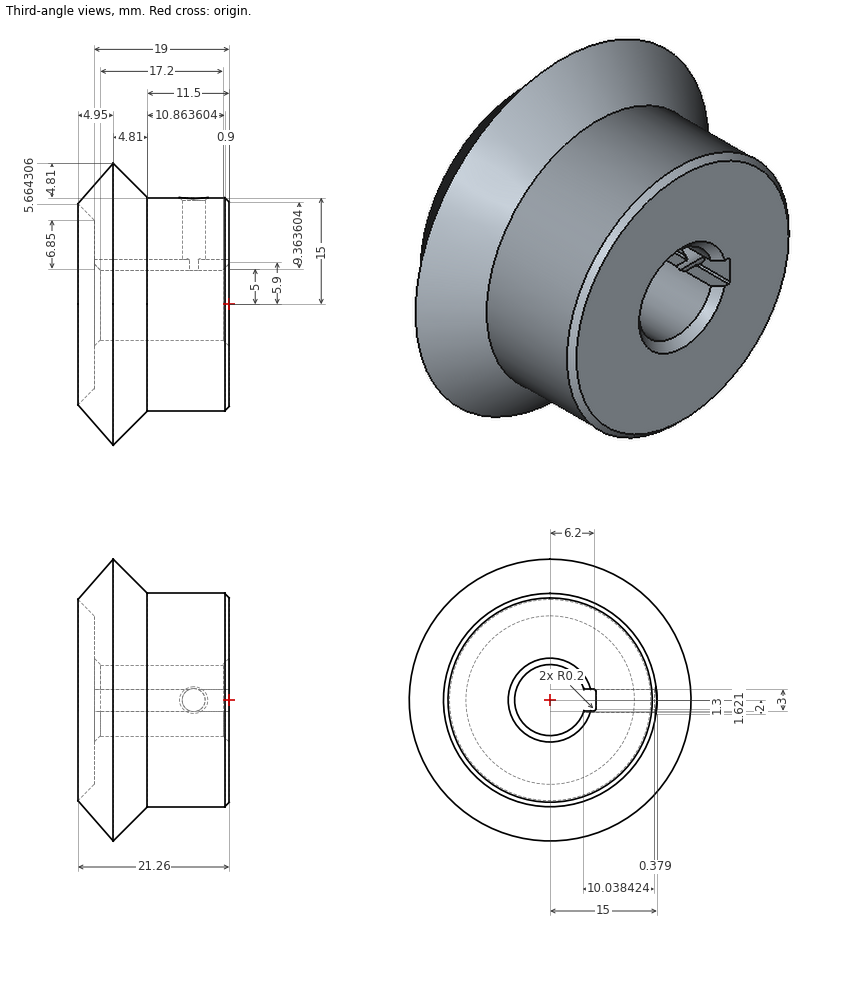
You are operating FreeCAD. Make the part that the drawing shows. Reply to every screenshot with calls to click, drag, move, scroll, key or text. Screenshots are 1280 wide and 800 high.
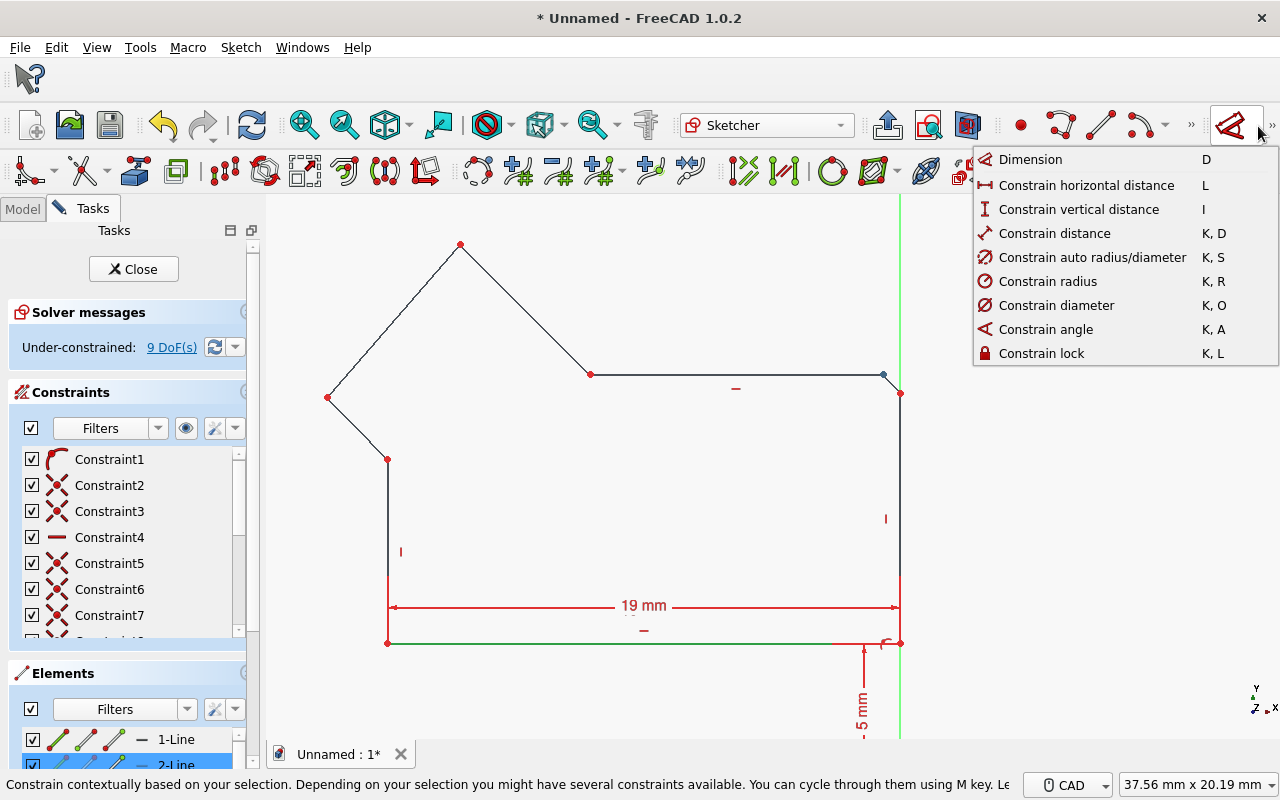
click(1126, 209)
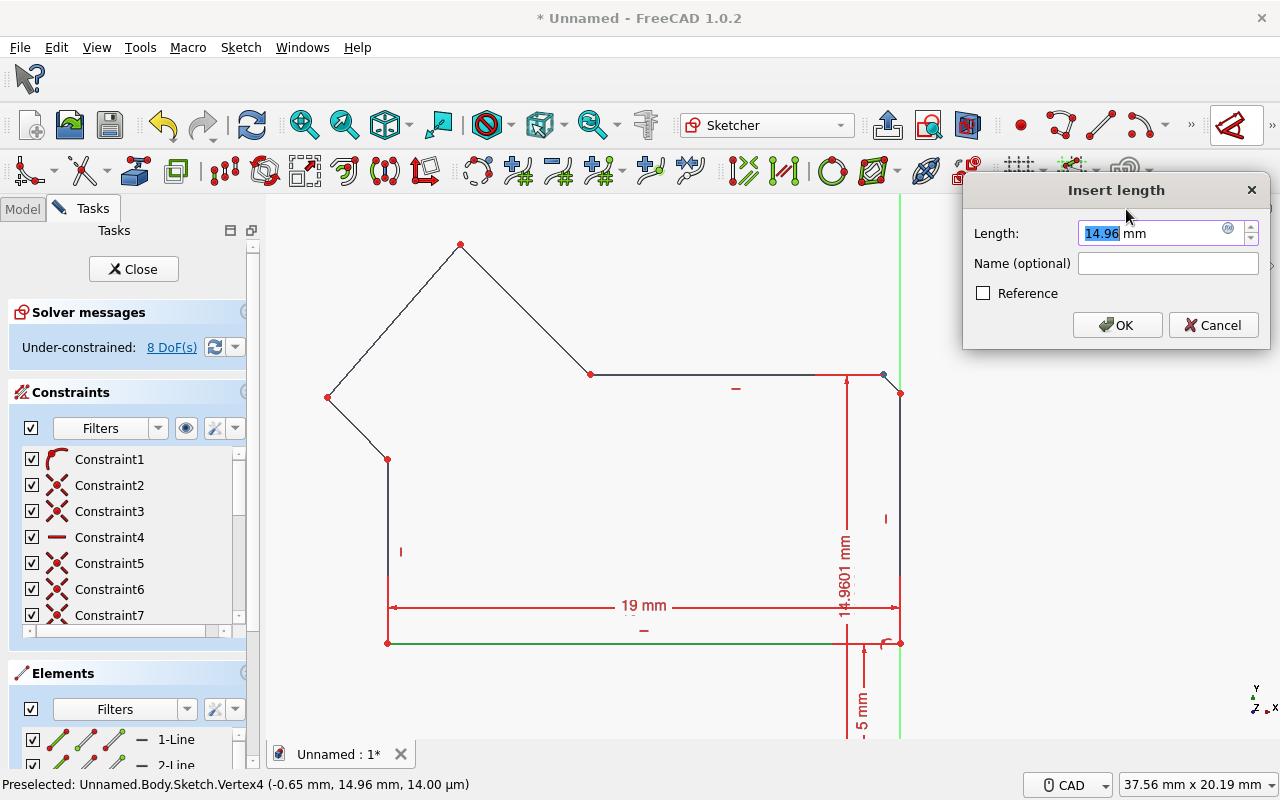
text(15)
key(Return)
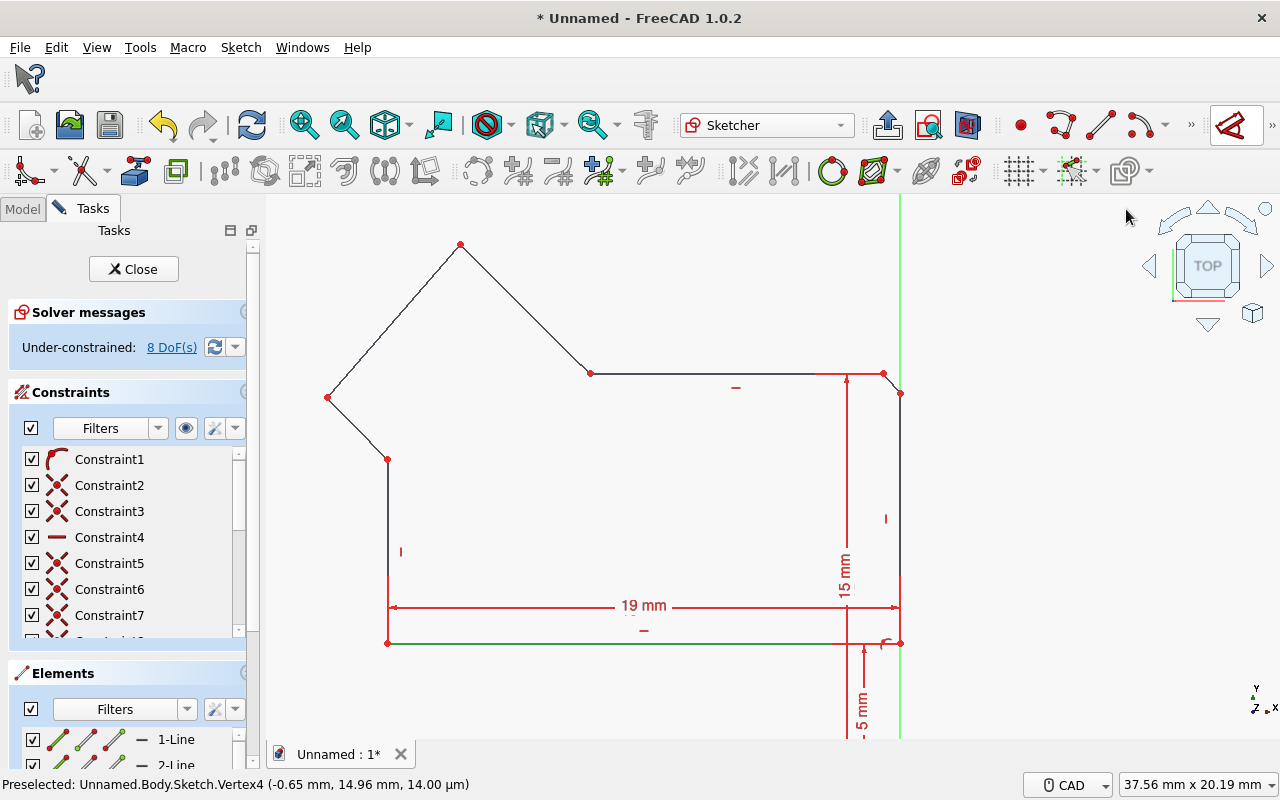
click(388, 515)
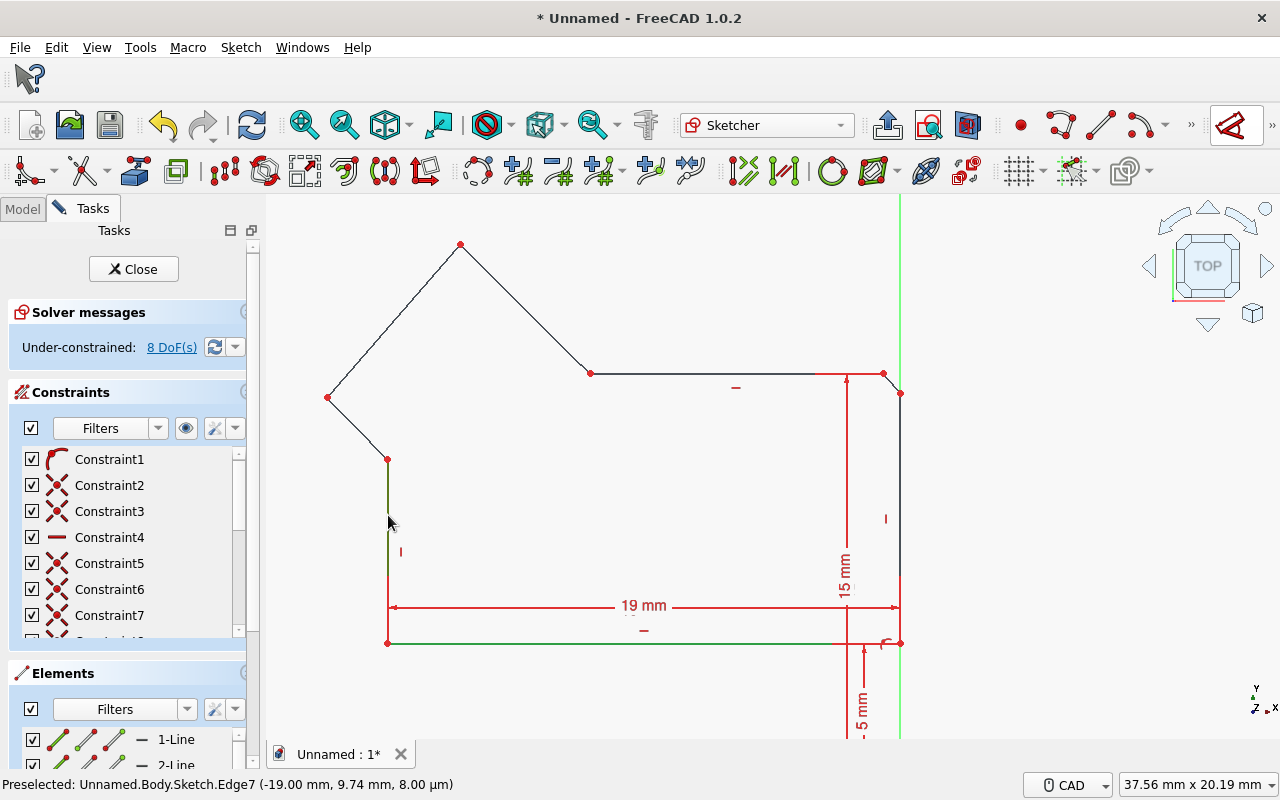
key(i)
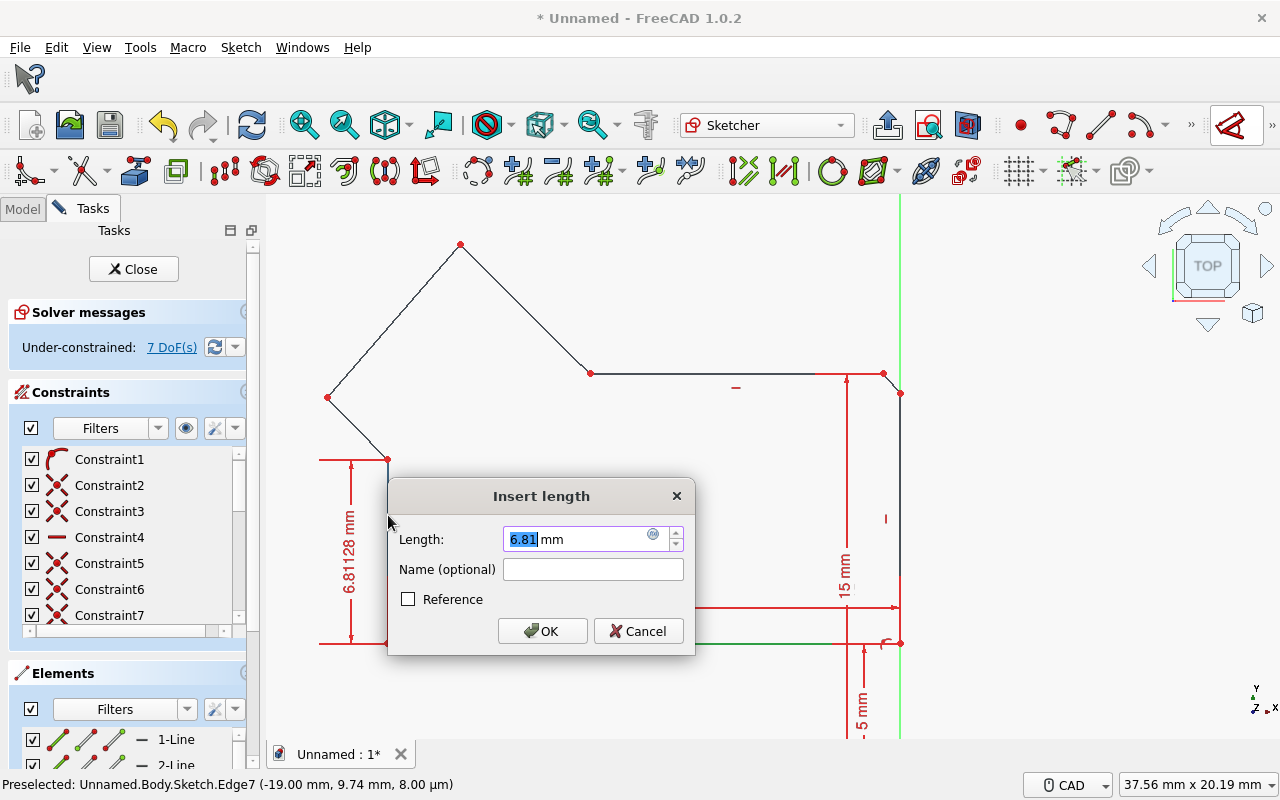
text(6.85)
key(Return)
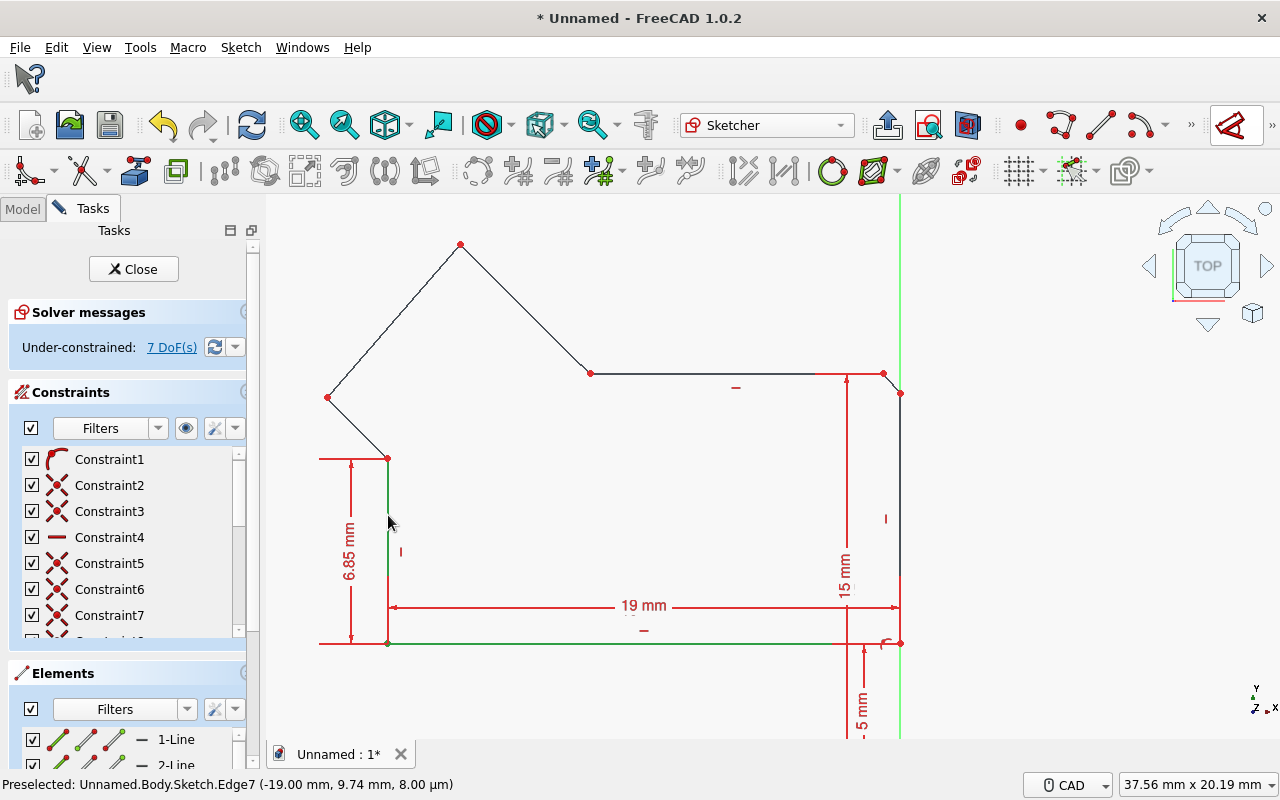
click(590, 374)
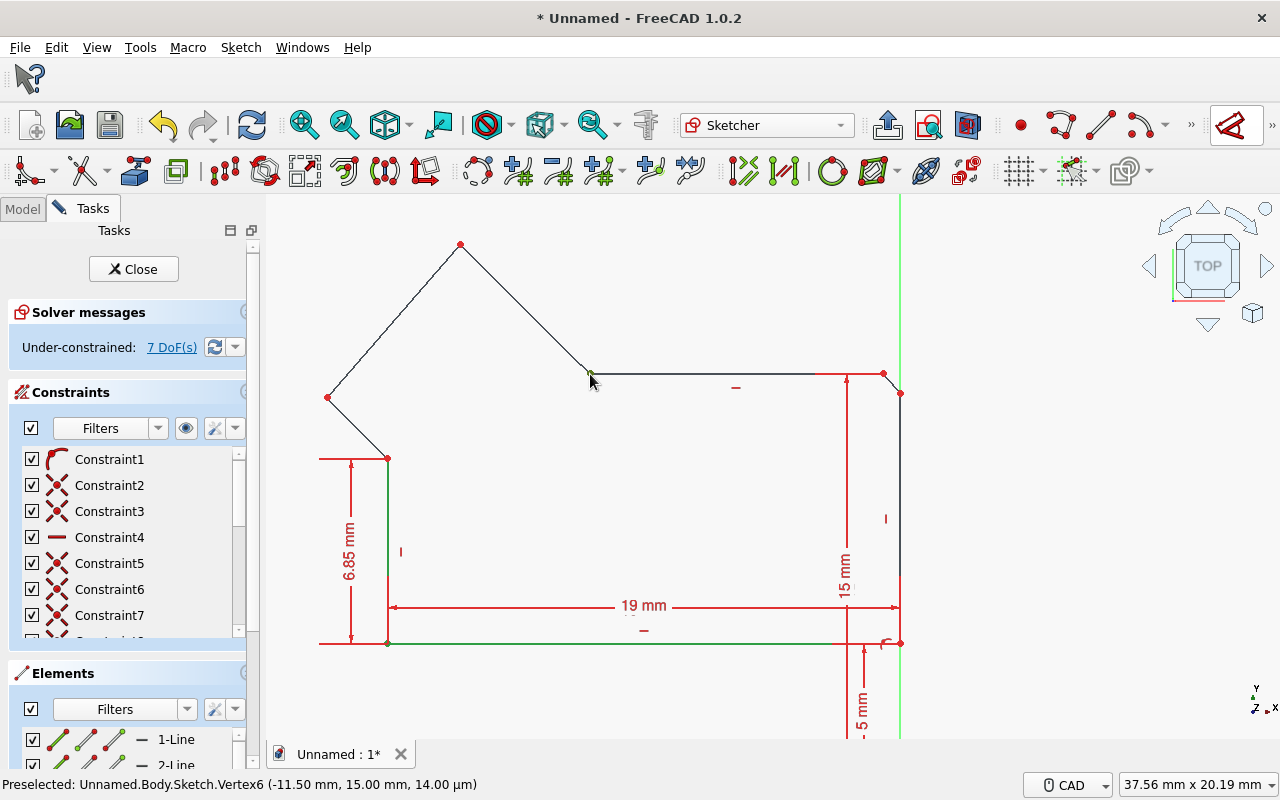
key(l)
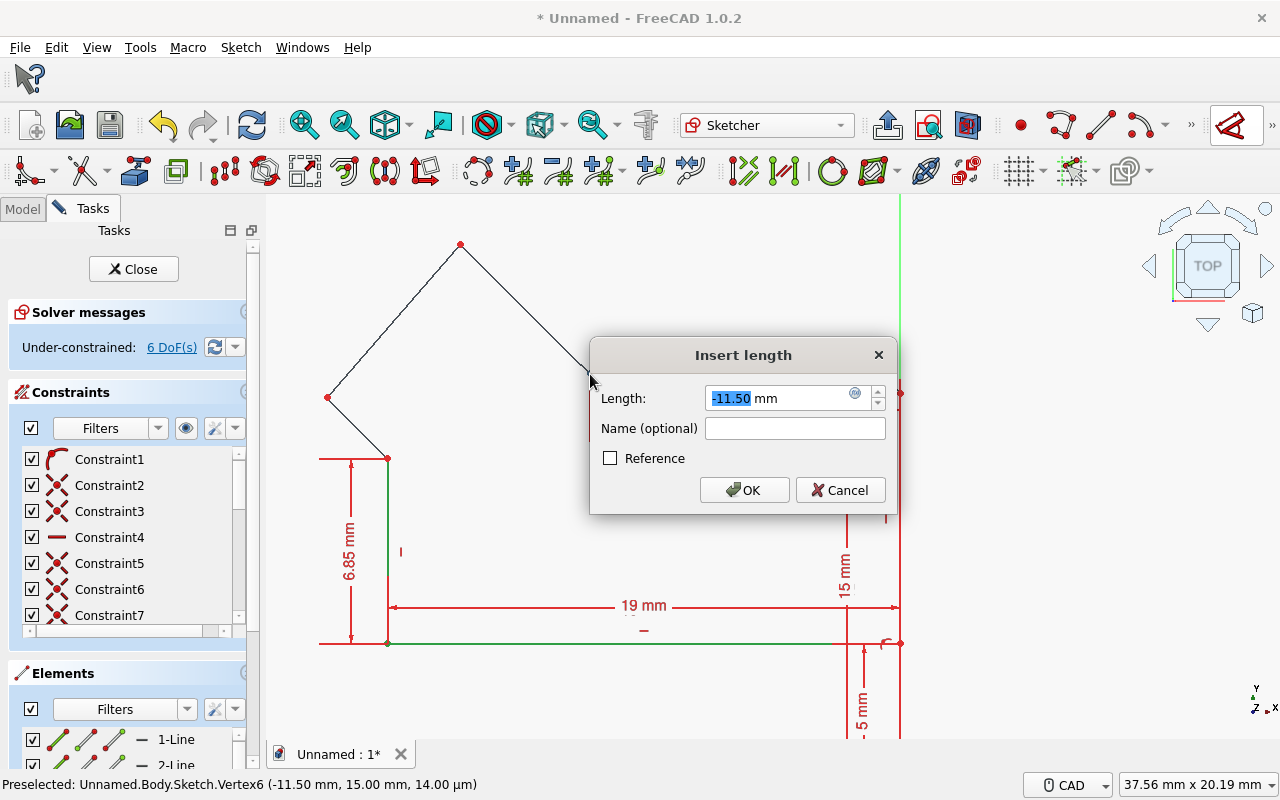
text(-11.5)
key(Return)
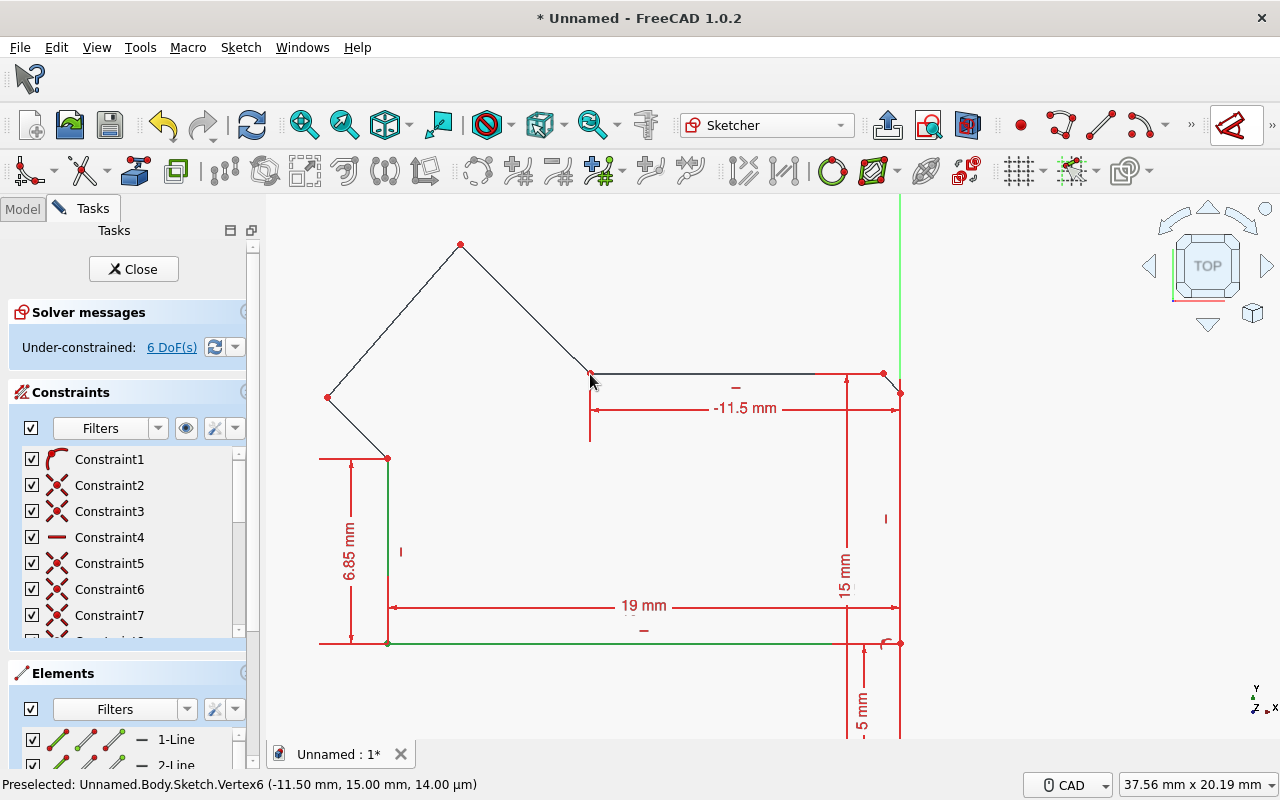
click(551, 335)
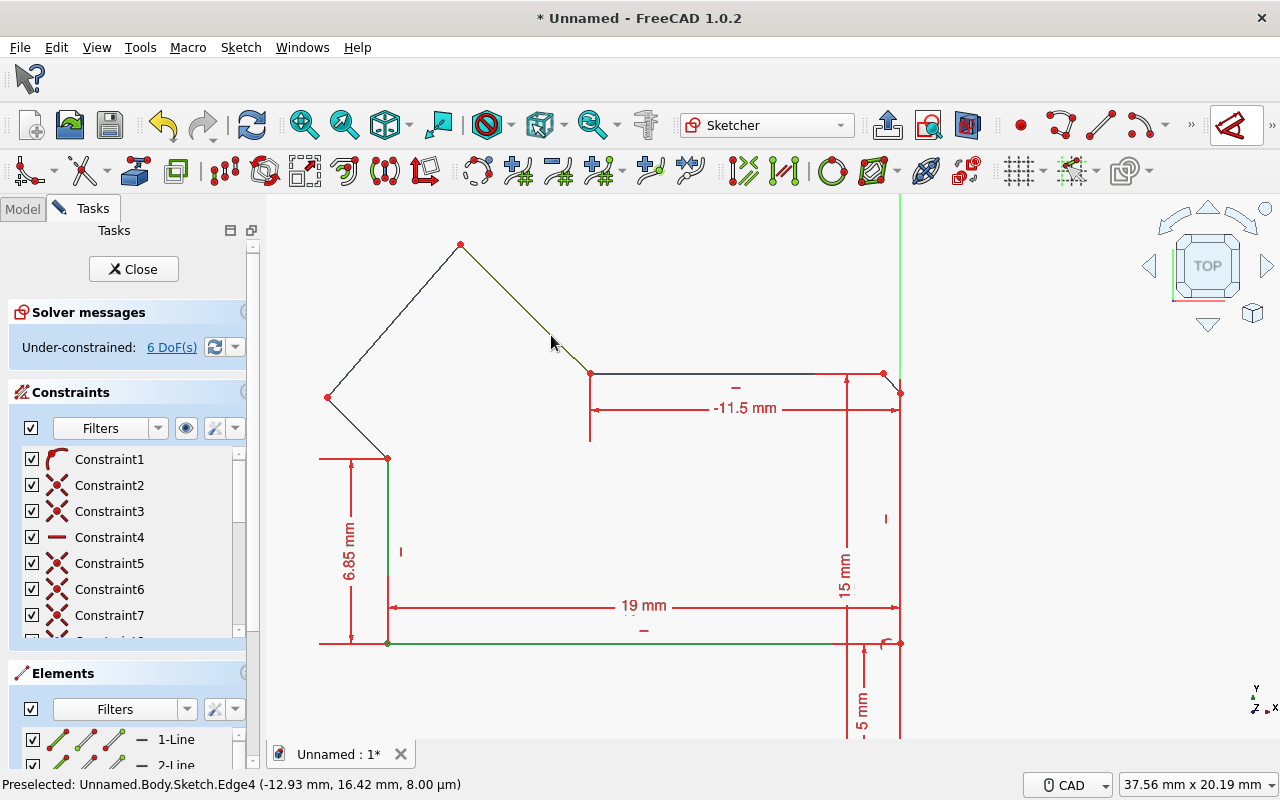
click(1258, 126)